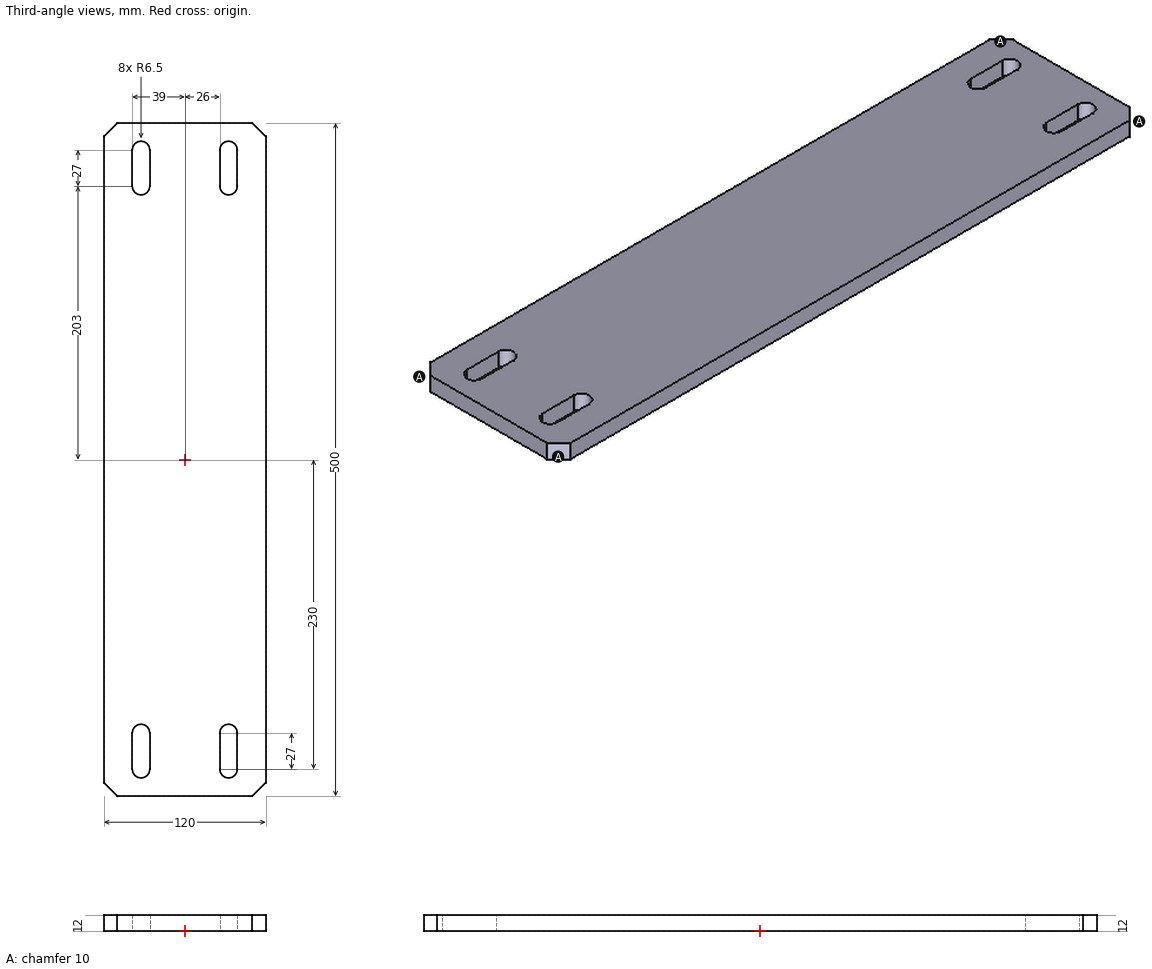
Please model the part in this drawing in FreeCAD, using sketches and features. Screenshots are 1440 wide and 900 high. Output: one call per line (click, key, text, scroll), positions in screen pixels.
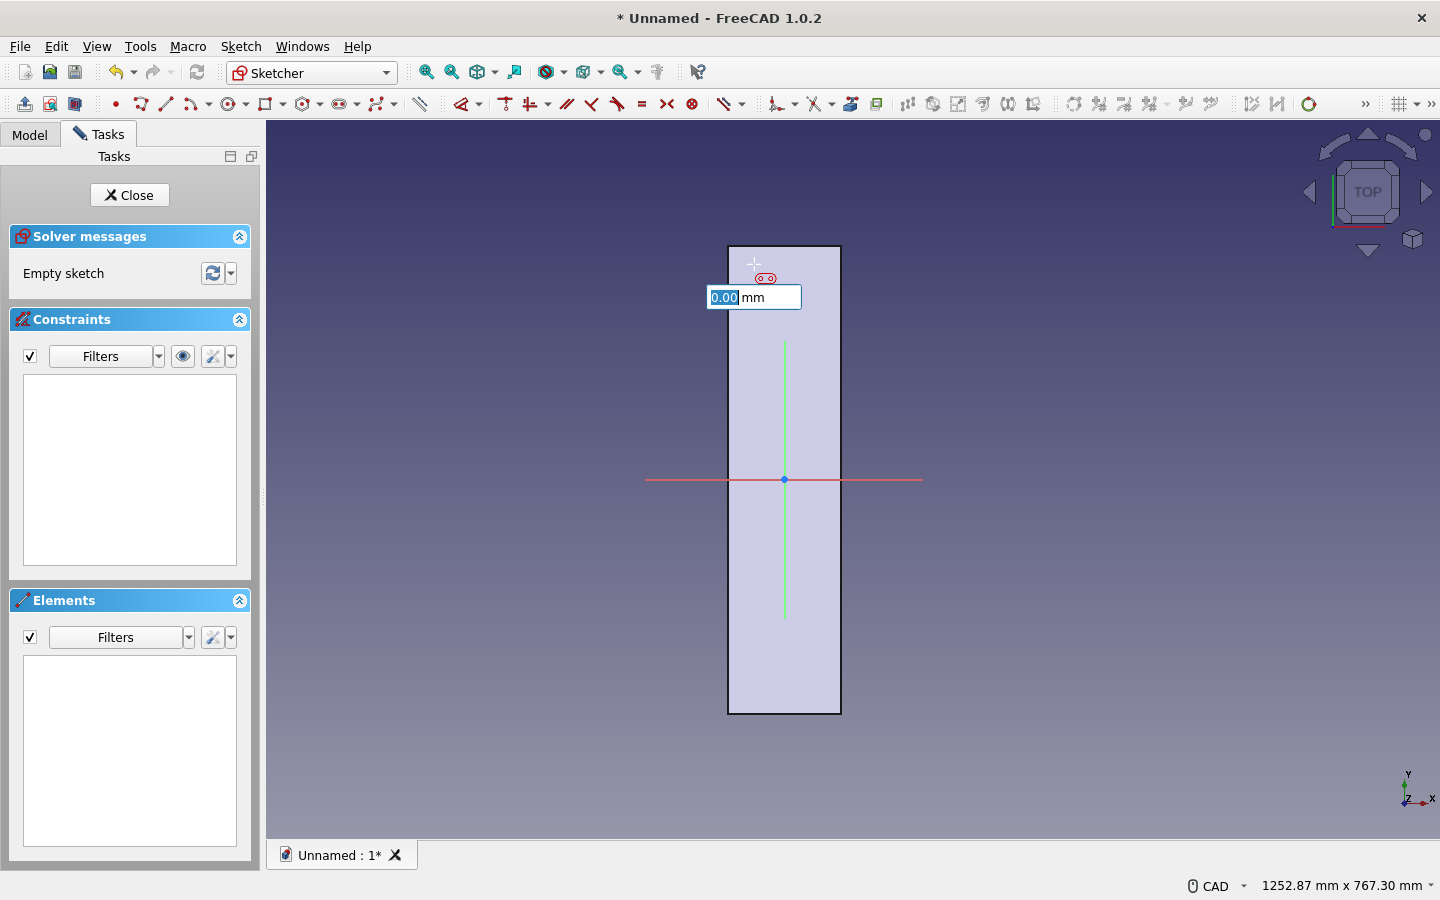
scroll(760, 277, up, 5)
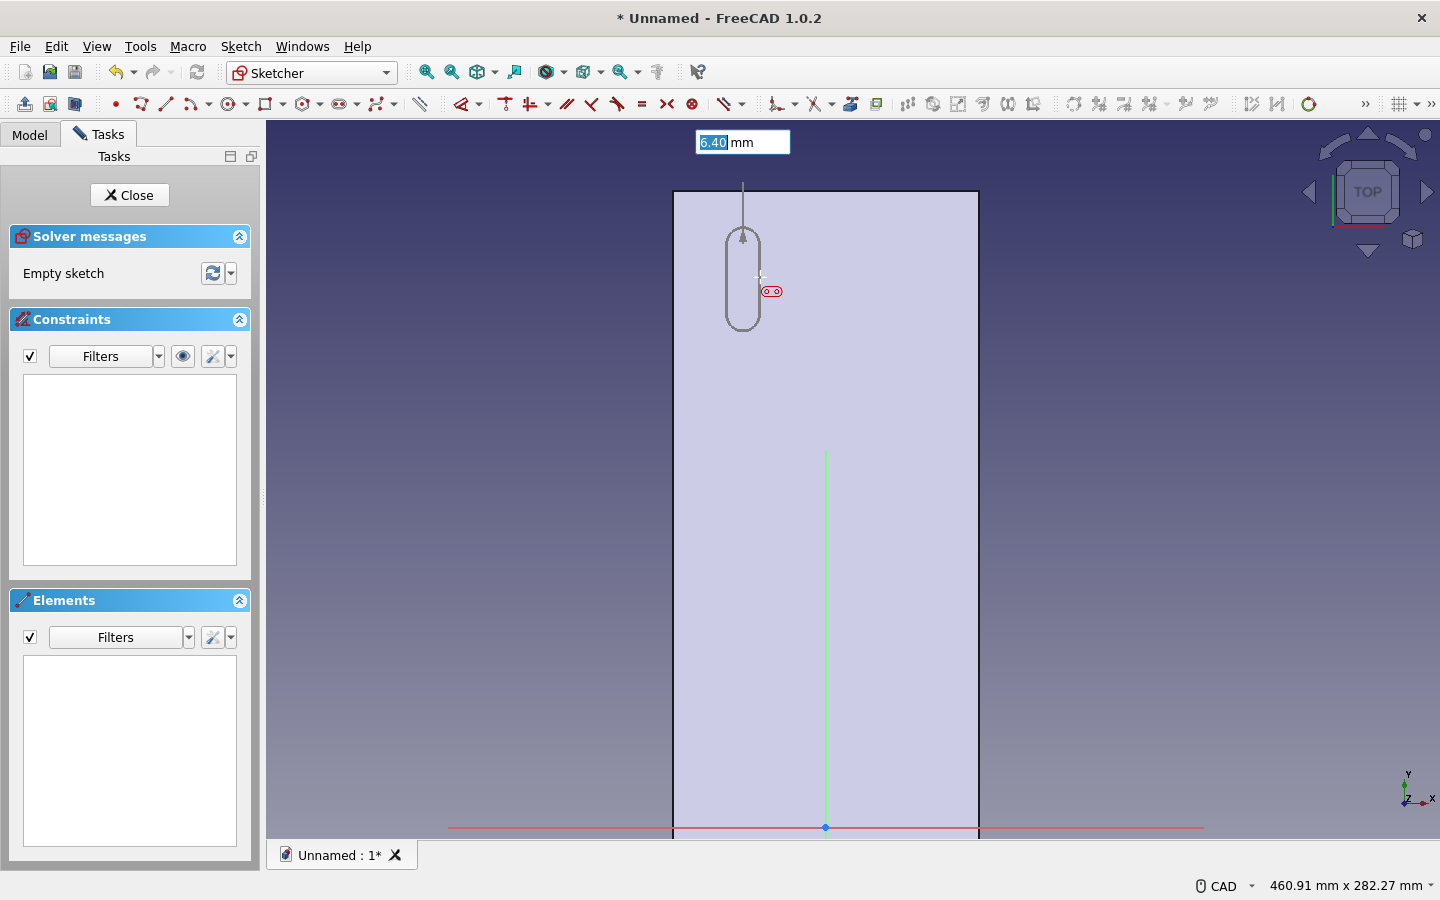
click(760, 277)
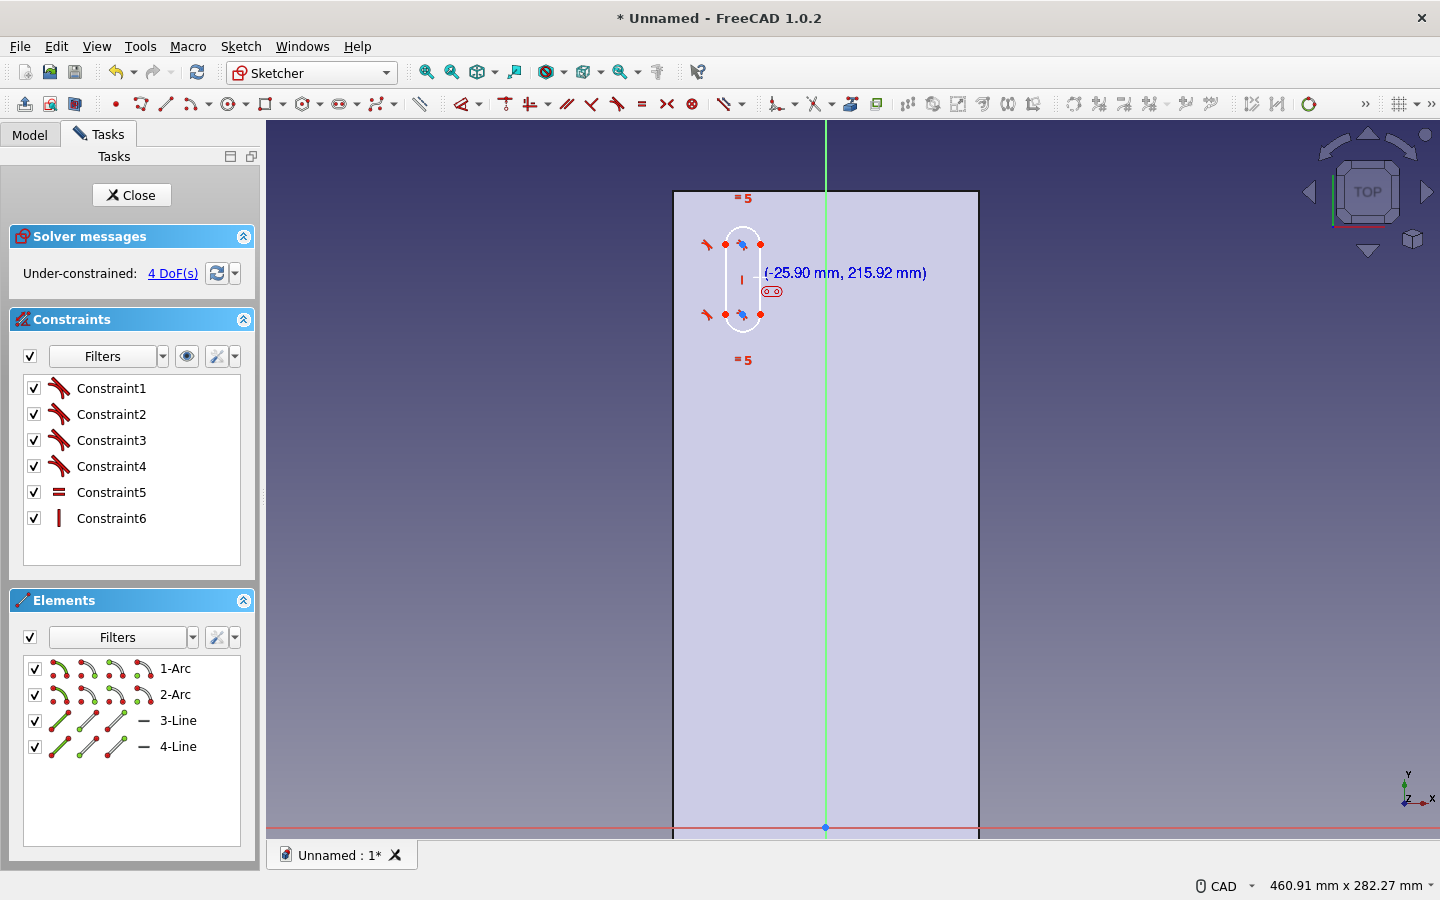
scroll(909, 311, up, 2)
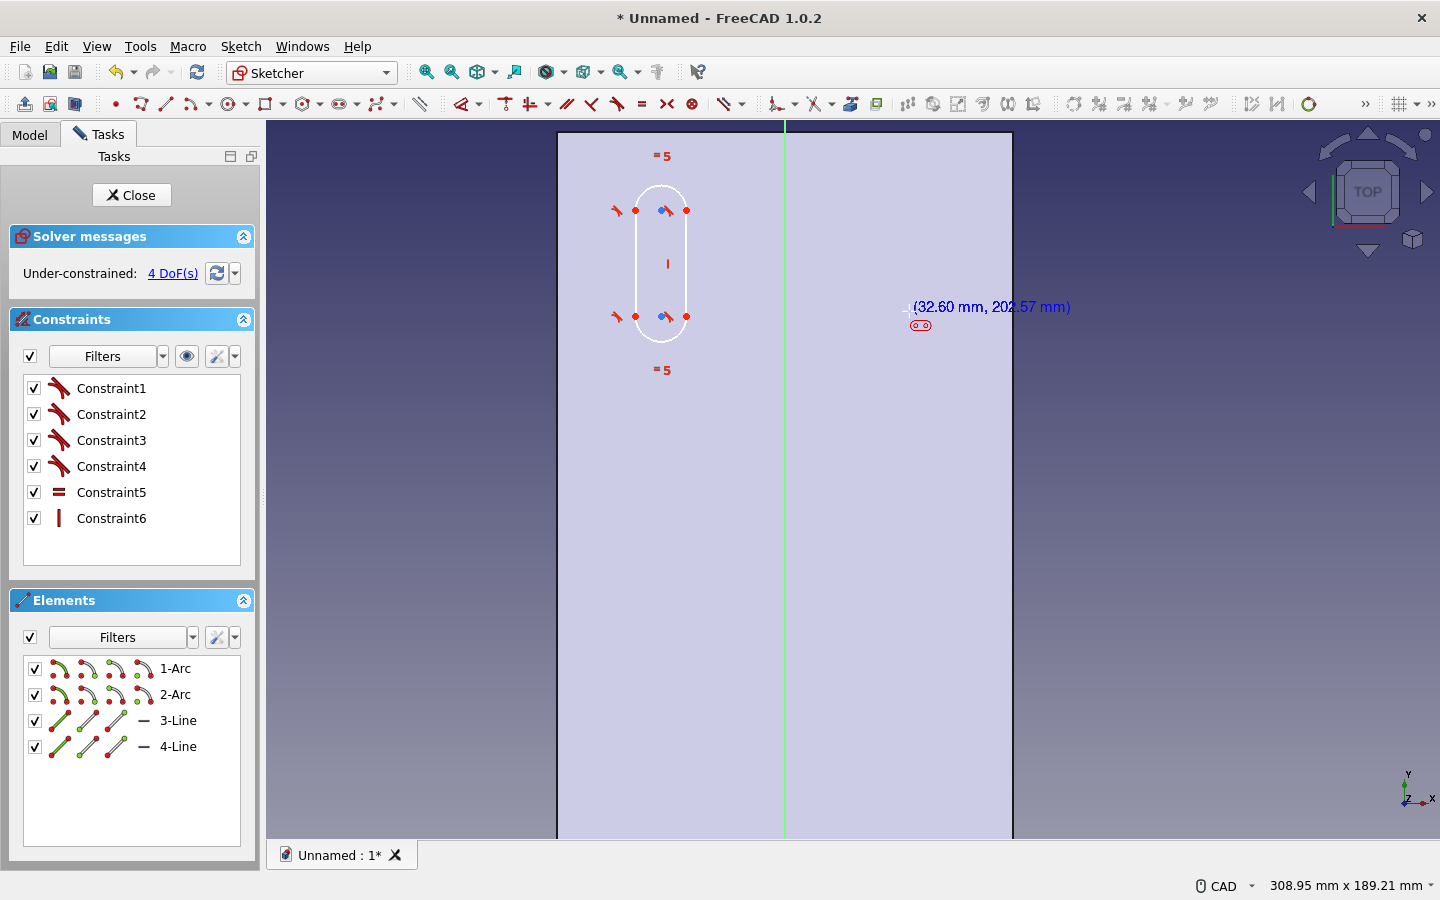
scroll(784, 282, down, 7)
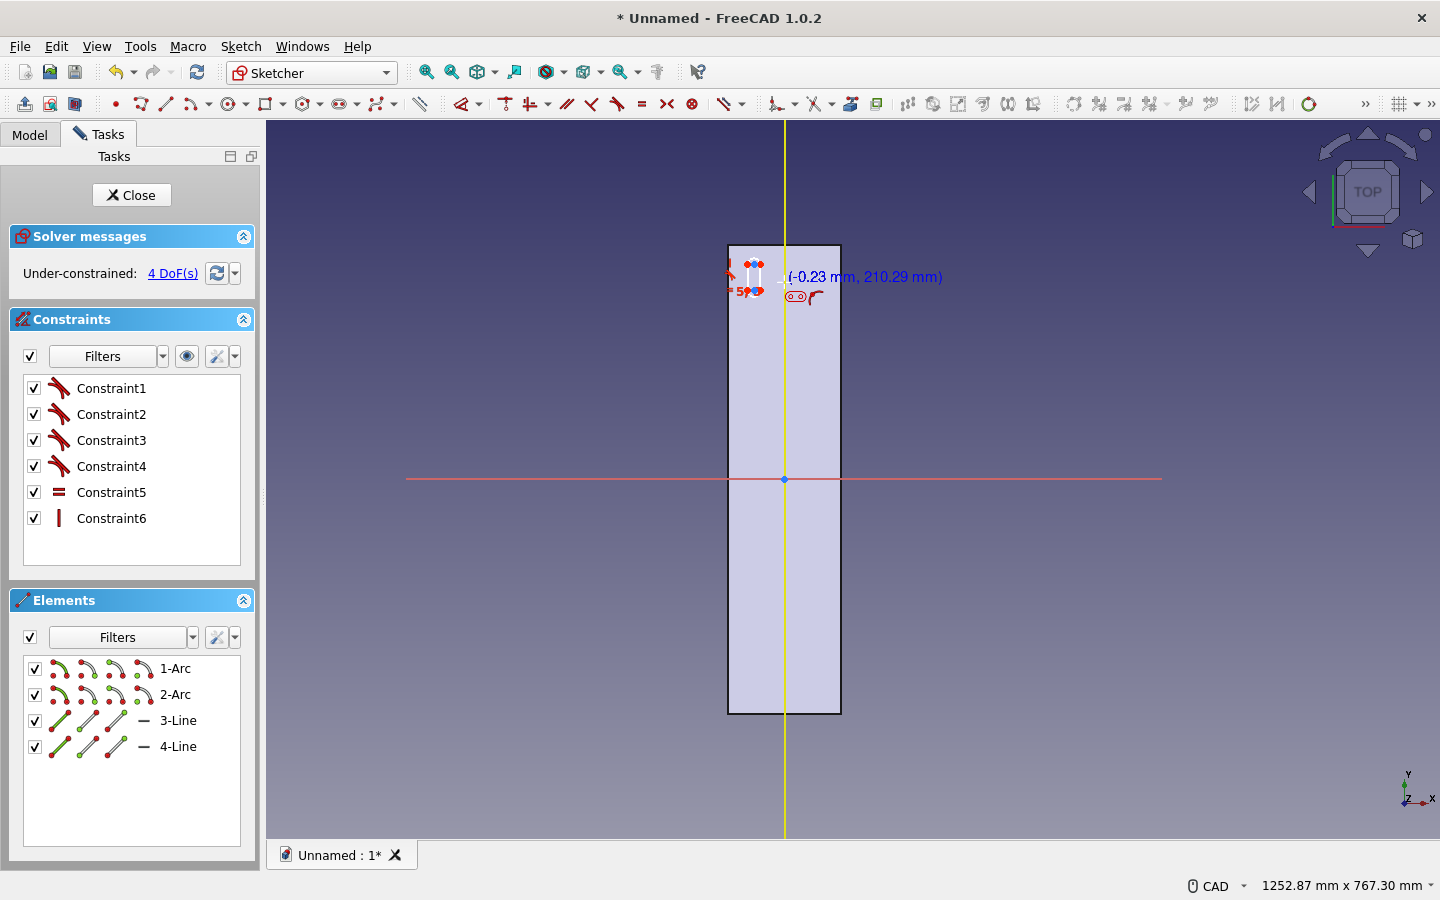
click(815, 289)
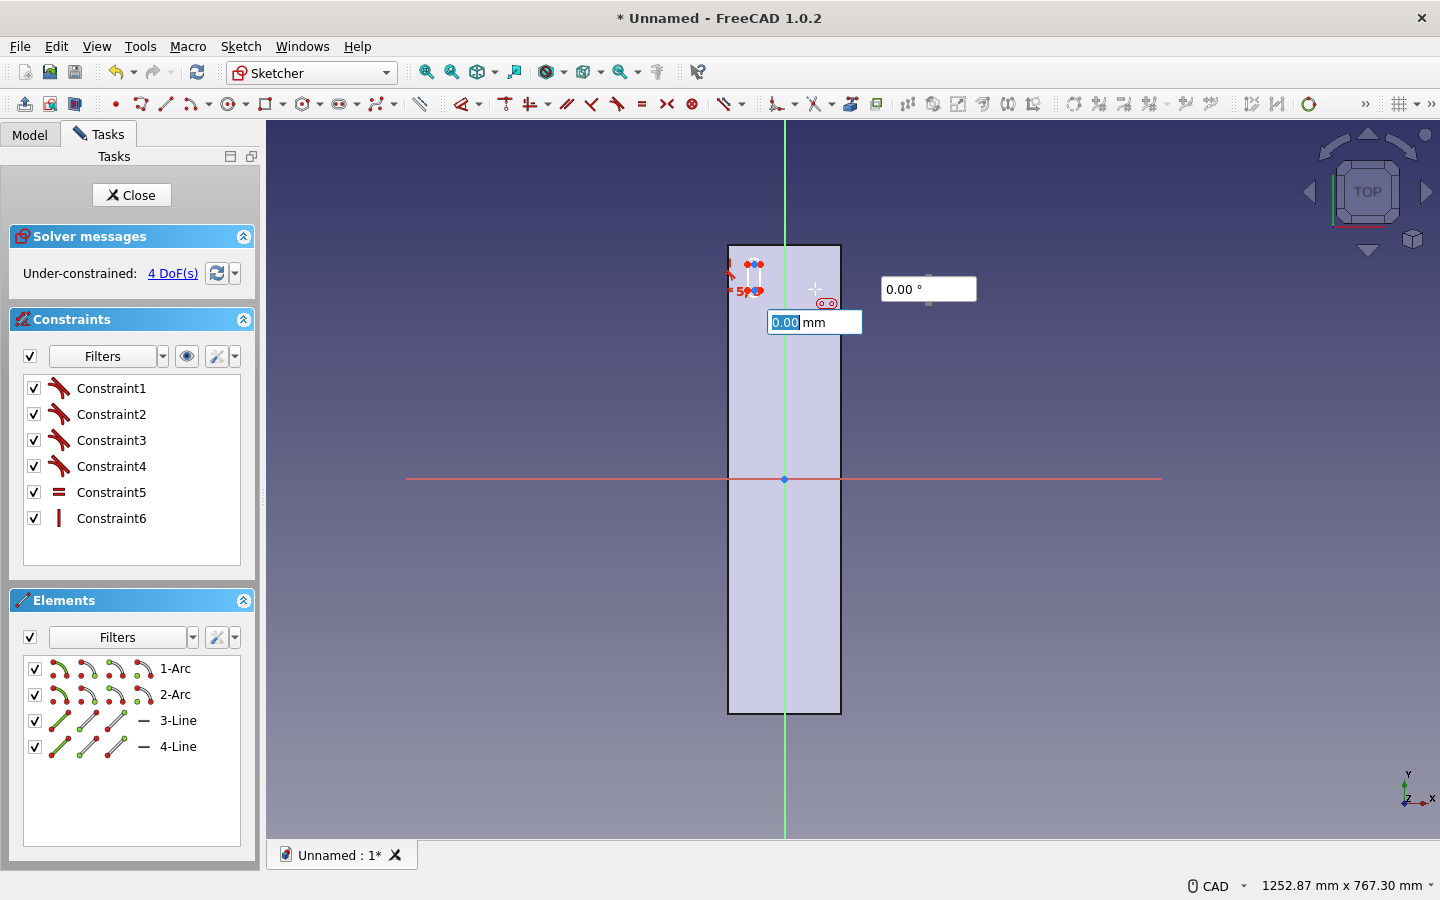
click(815, 264)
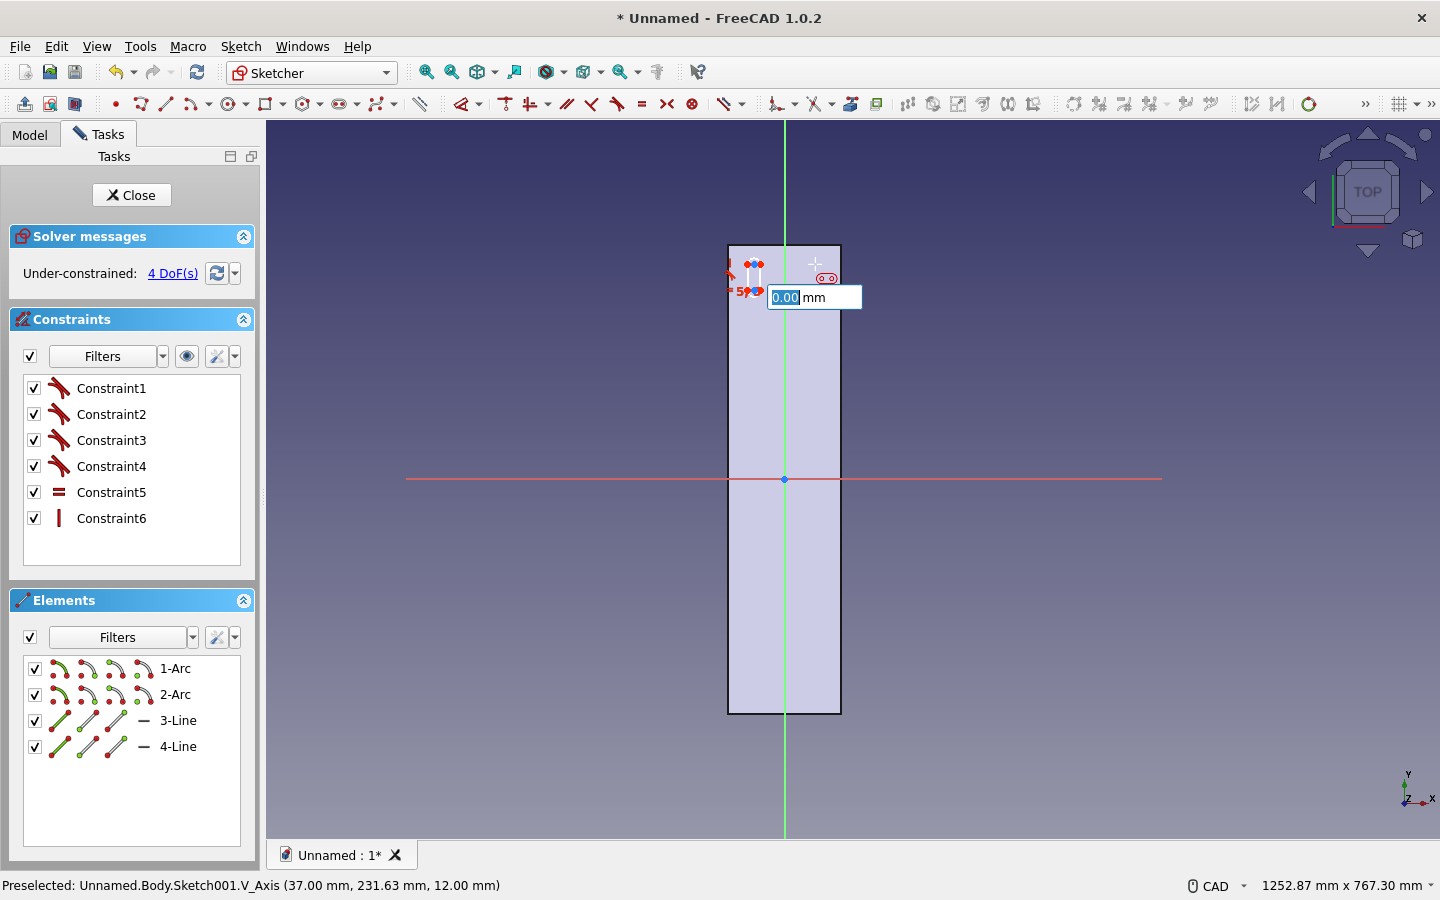
scroll(809, 277, up, 5)